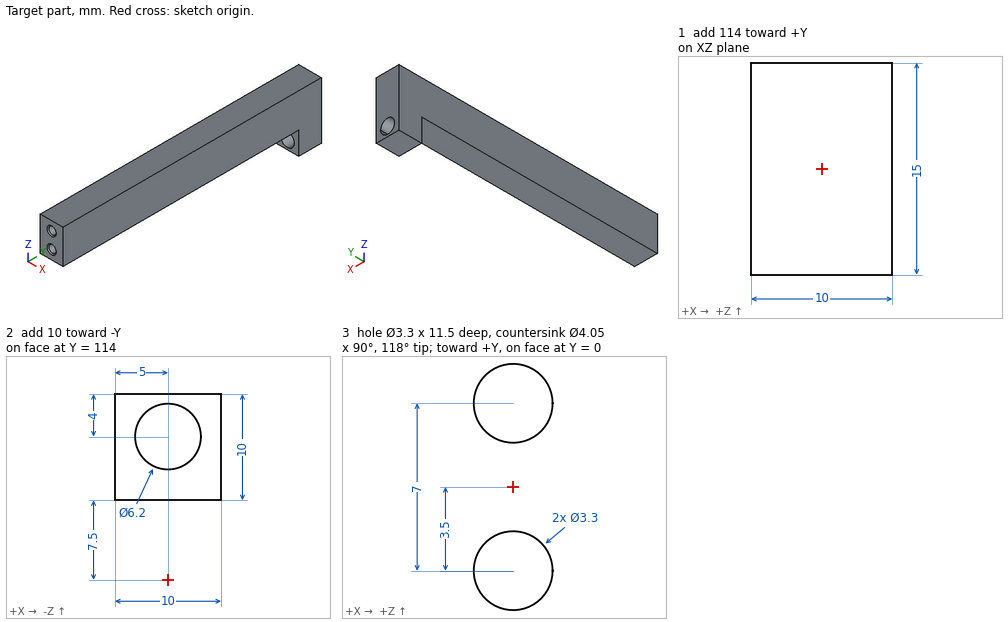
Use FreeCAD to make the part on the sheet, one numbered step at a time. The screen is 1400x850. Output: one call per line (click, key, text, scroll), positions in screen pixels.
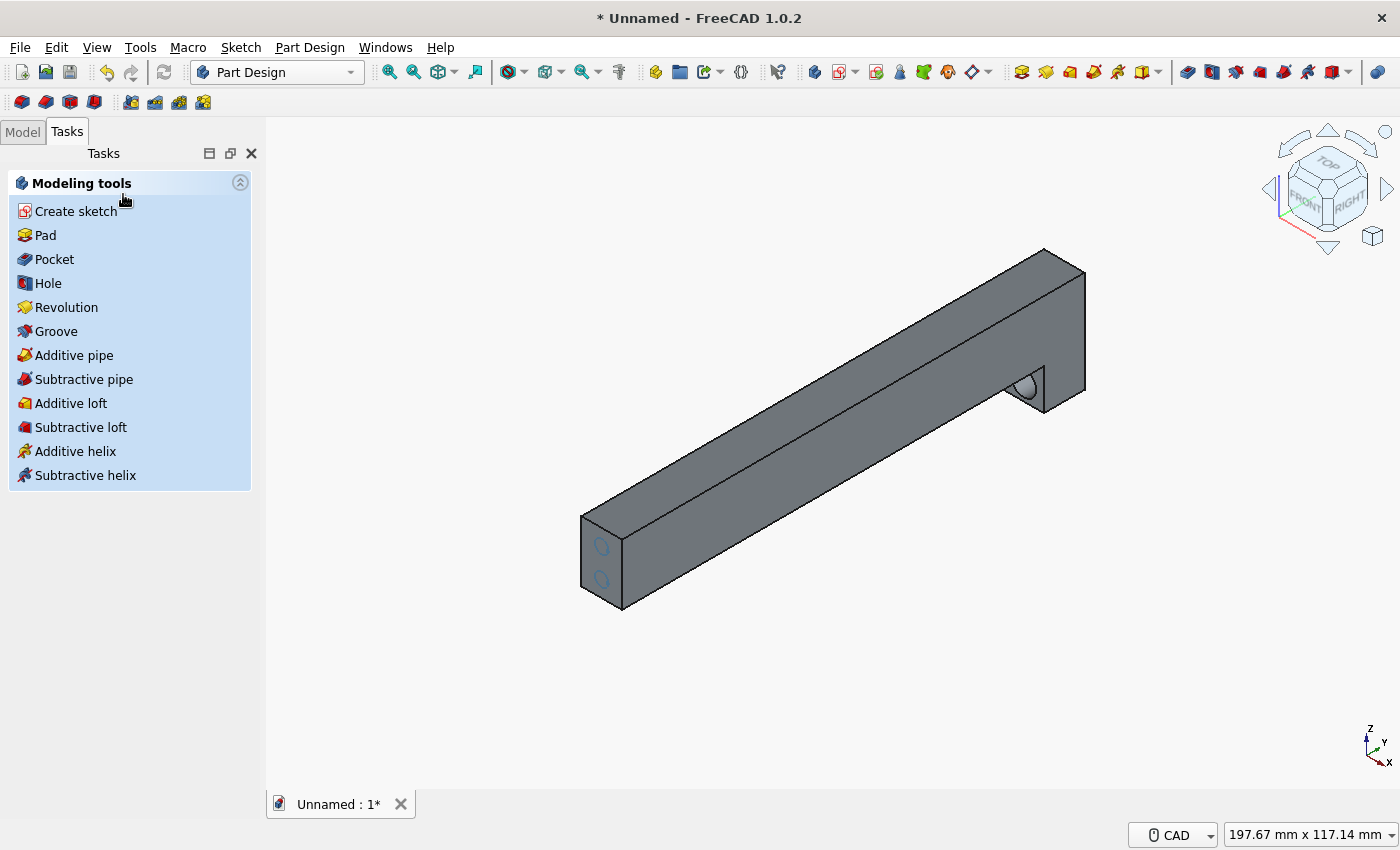
click(1212, 72)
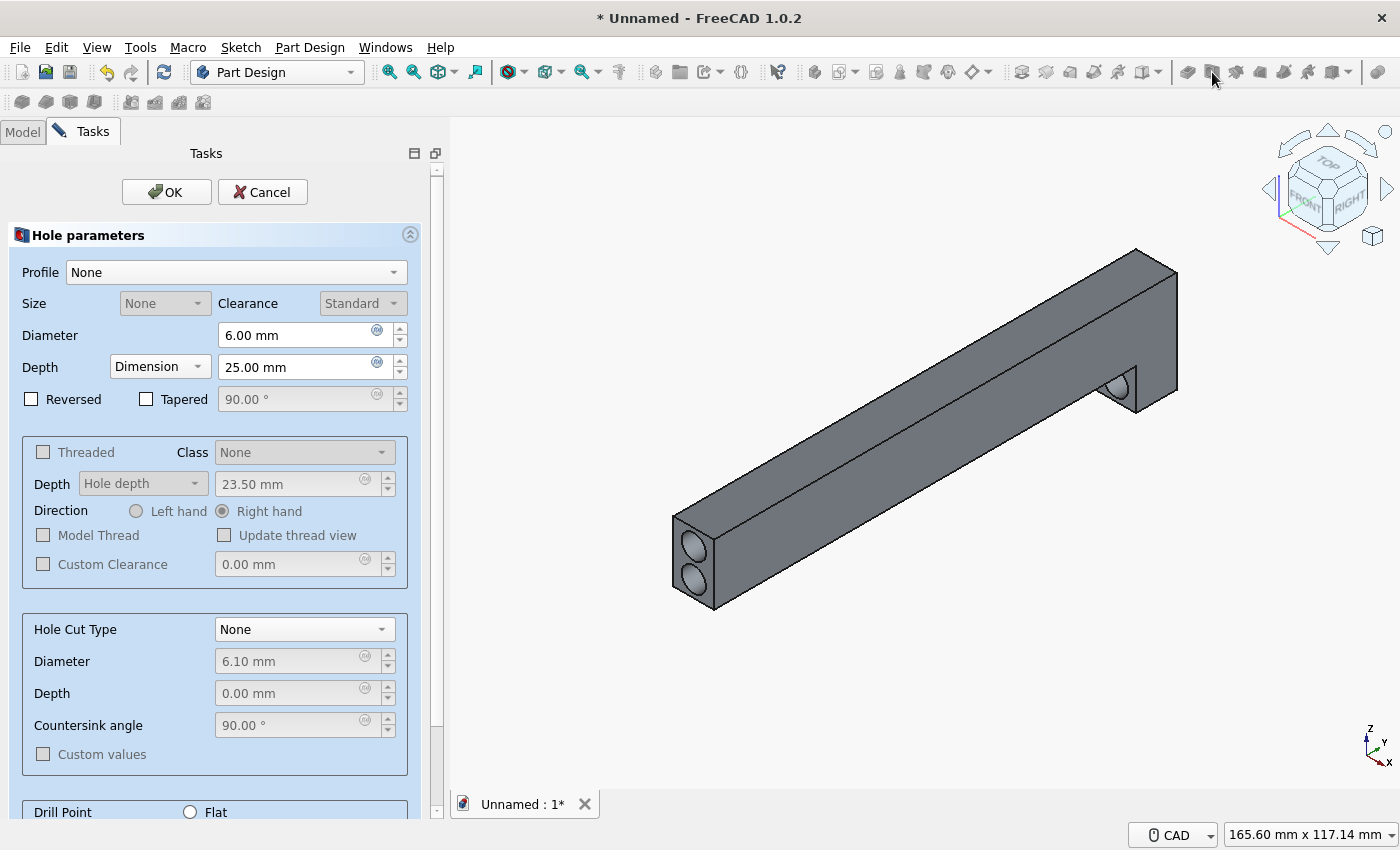
triple_click(305, 335)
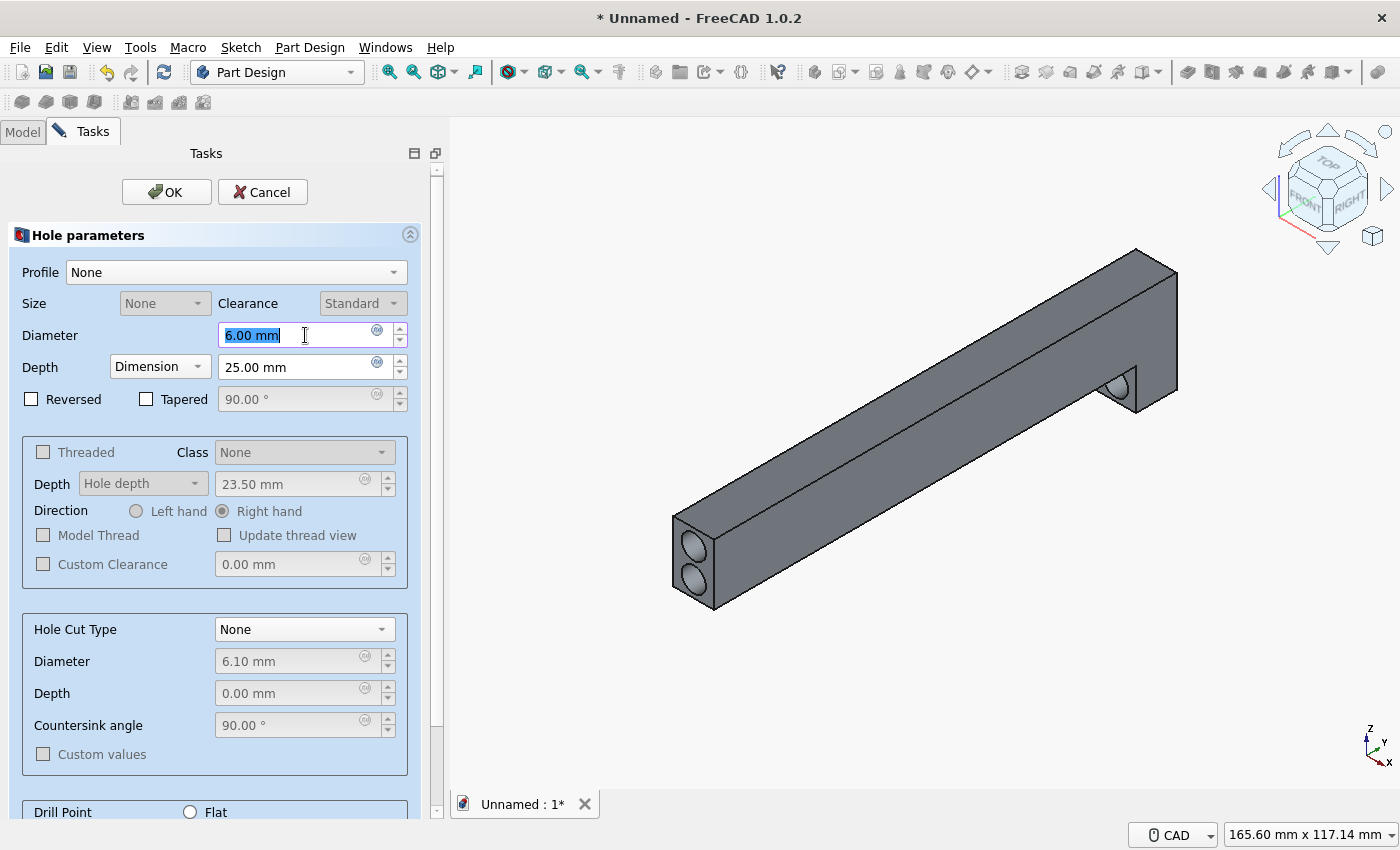
text(3.3)
key(Tab)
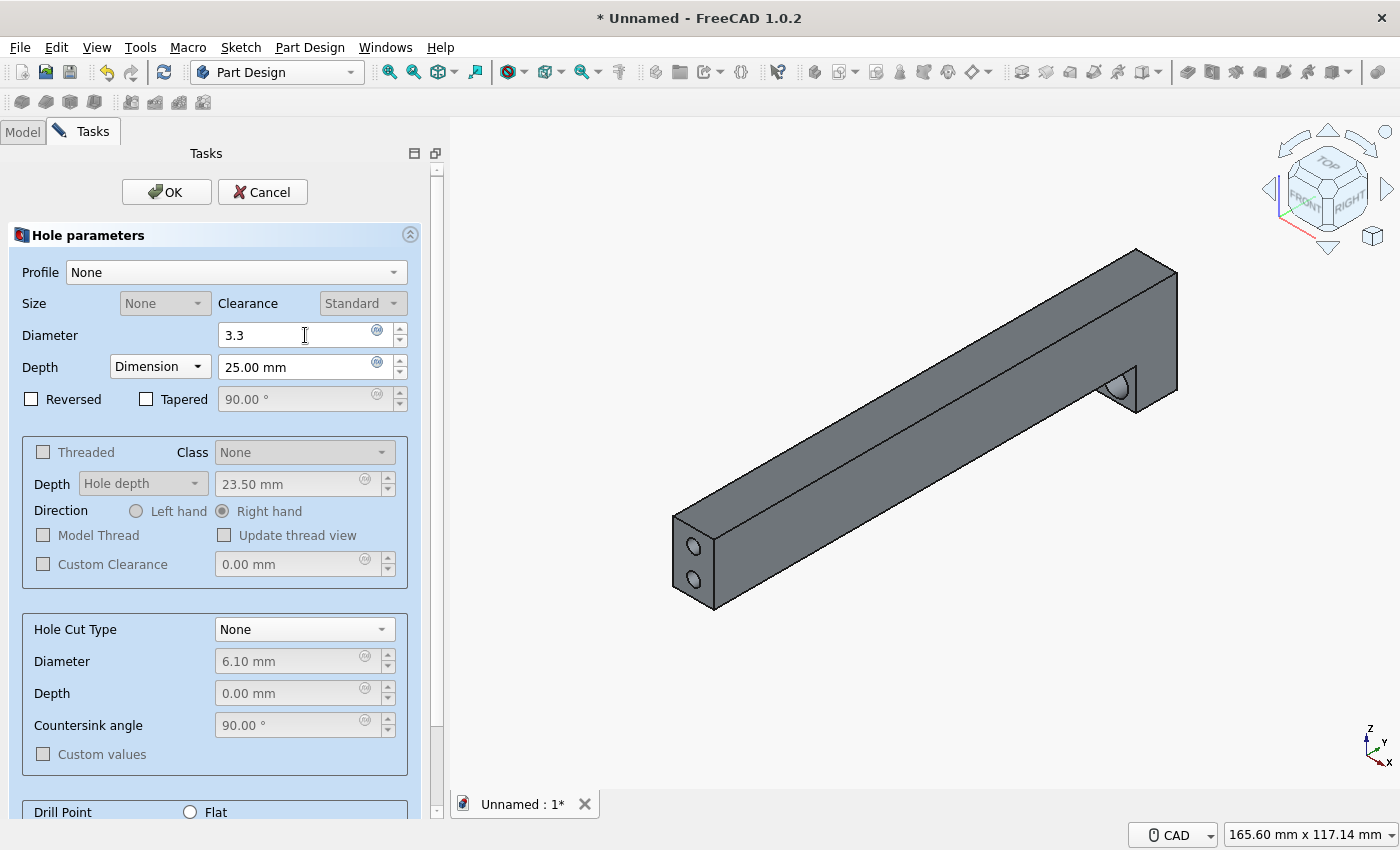
triple_click(305, 367)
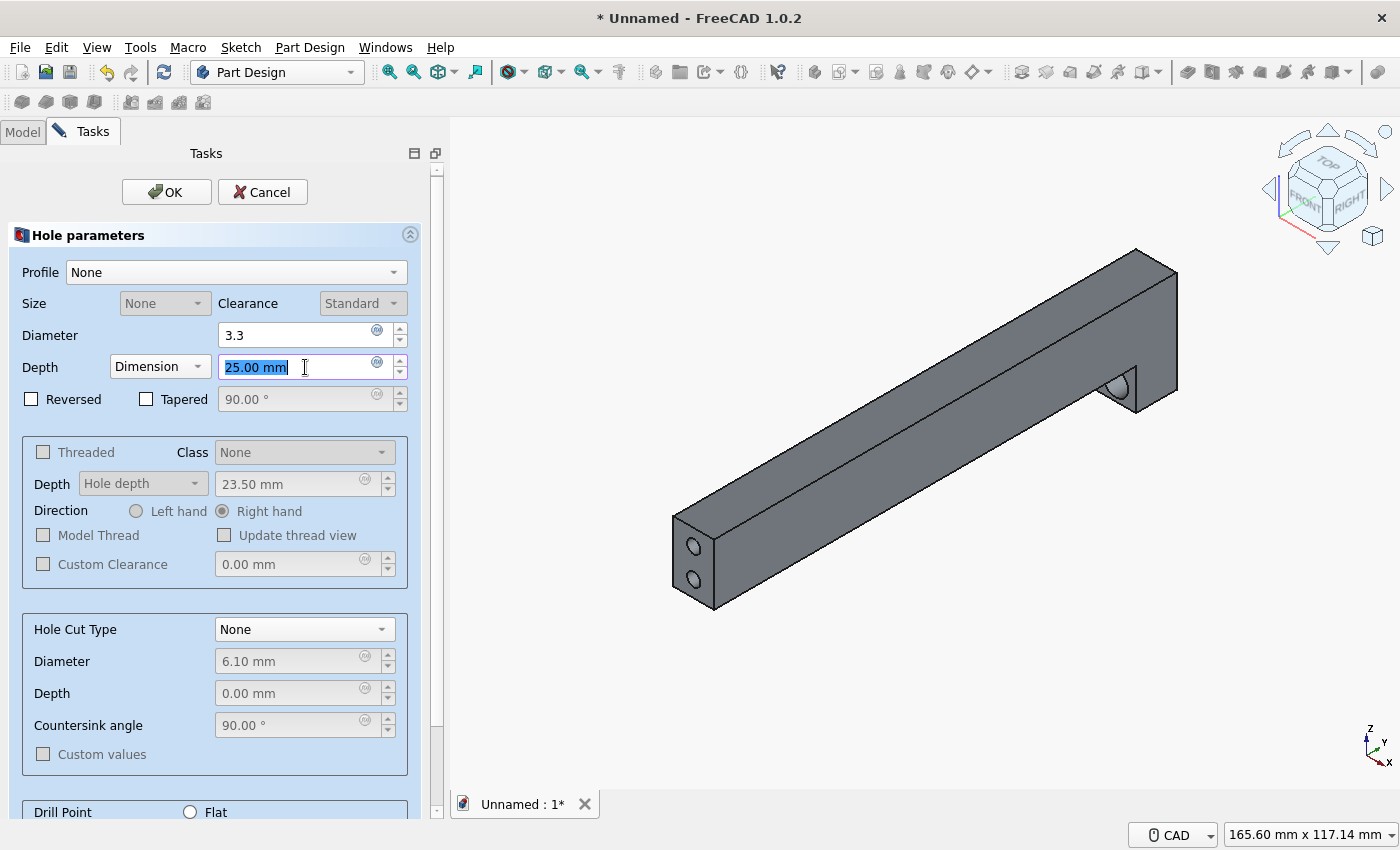
text(11.5)
key(Tab)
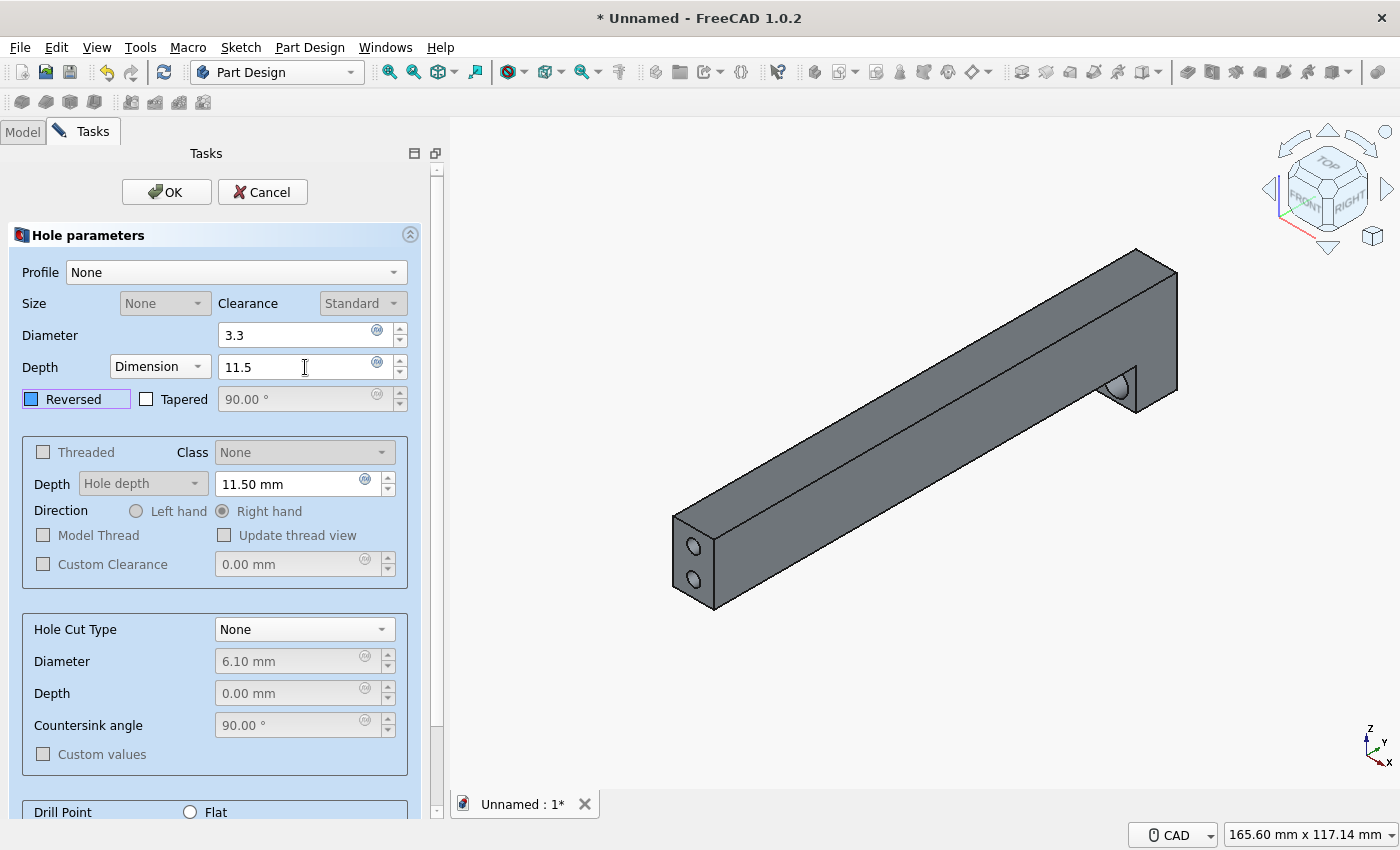
click(306, 630)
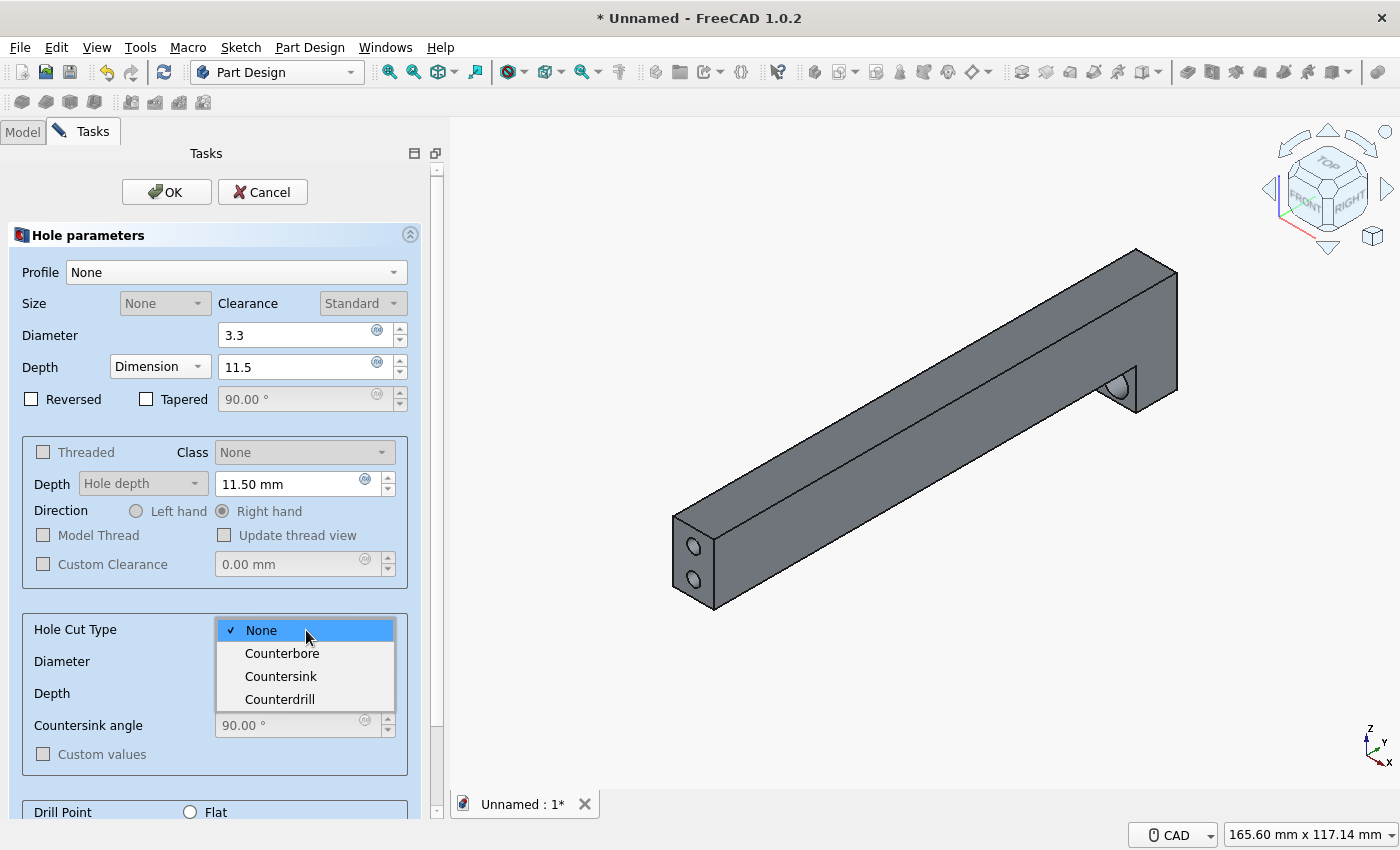
click(304, 676)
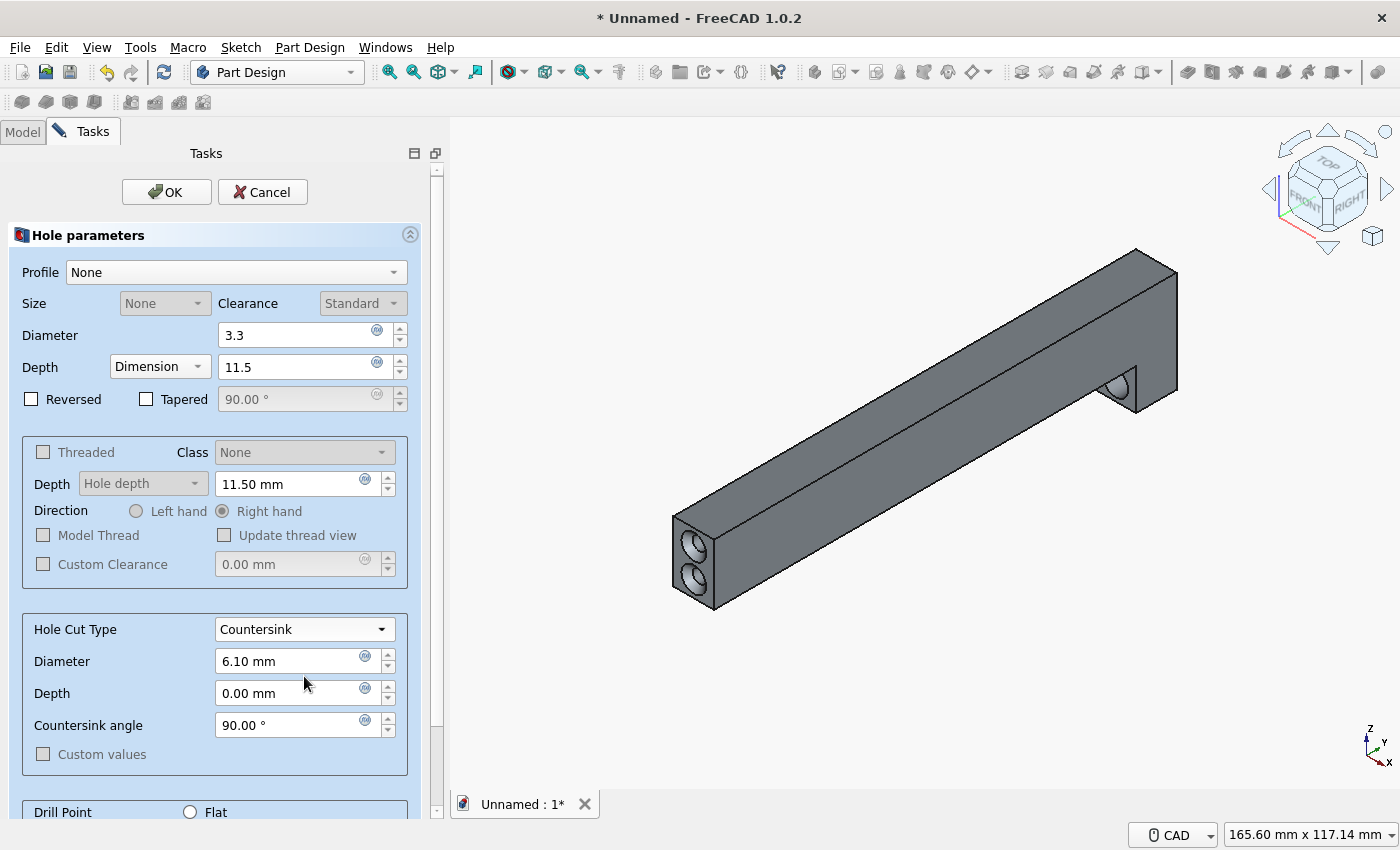
triple_click(298, 661)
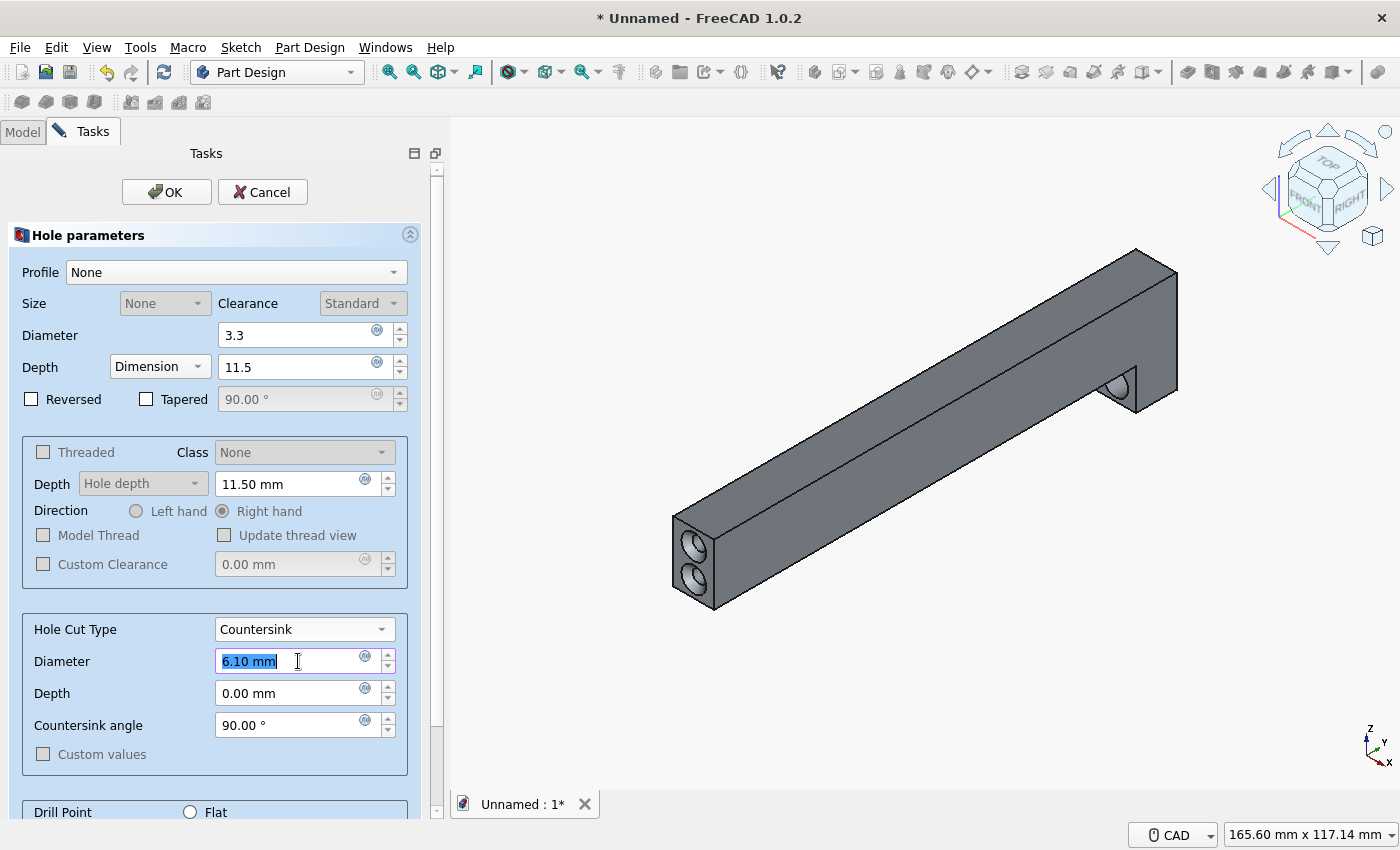
text(4.05)
key(Tab)